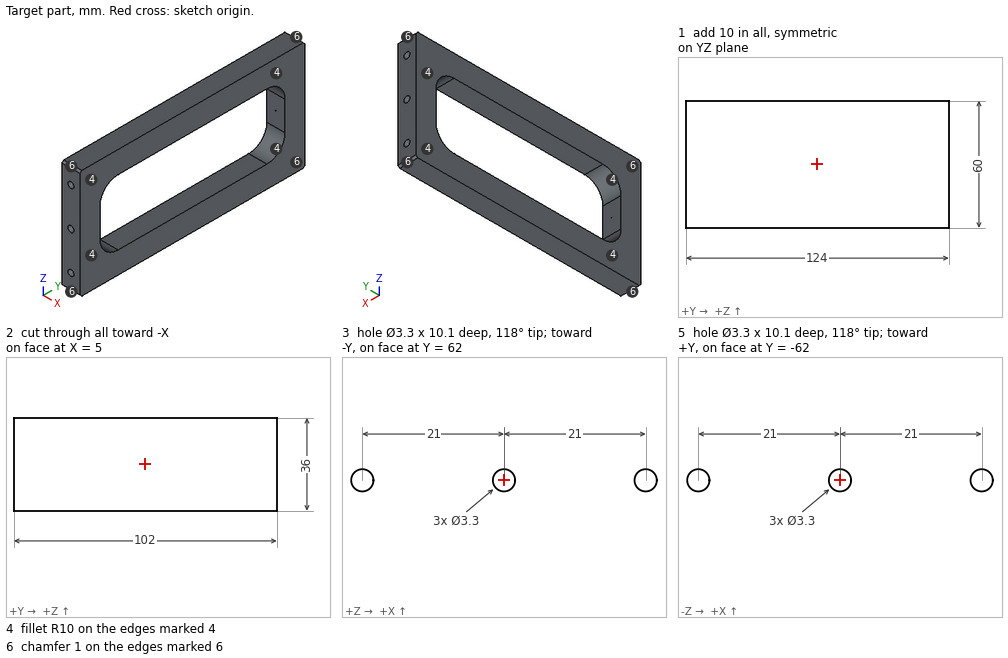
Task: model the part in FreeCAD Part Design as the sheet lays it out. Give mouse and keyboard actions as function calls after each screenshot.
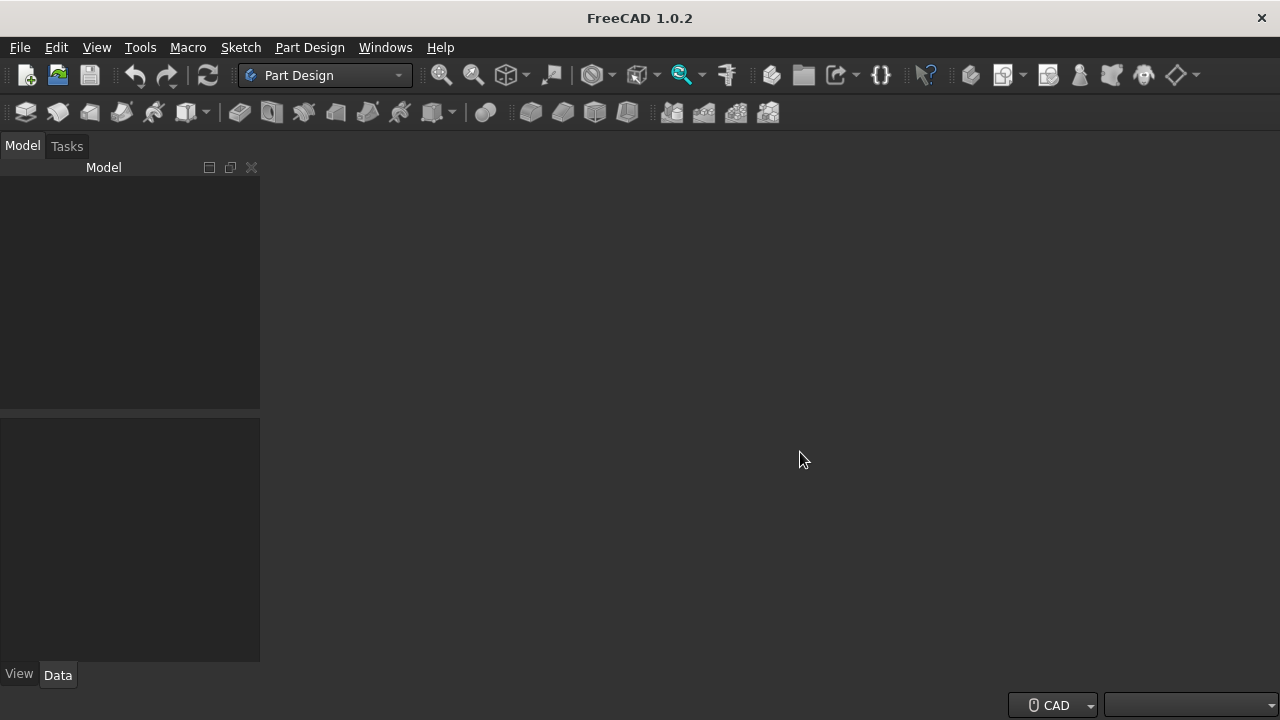
key(ctrl+n)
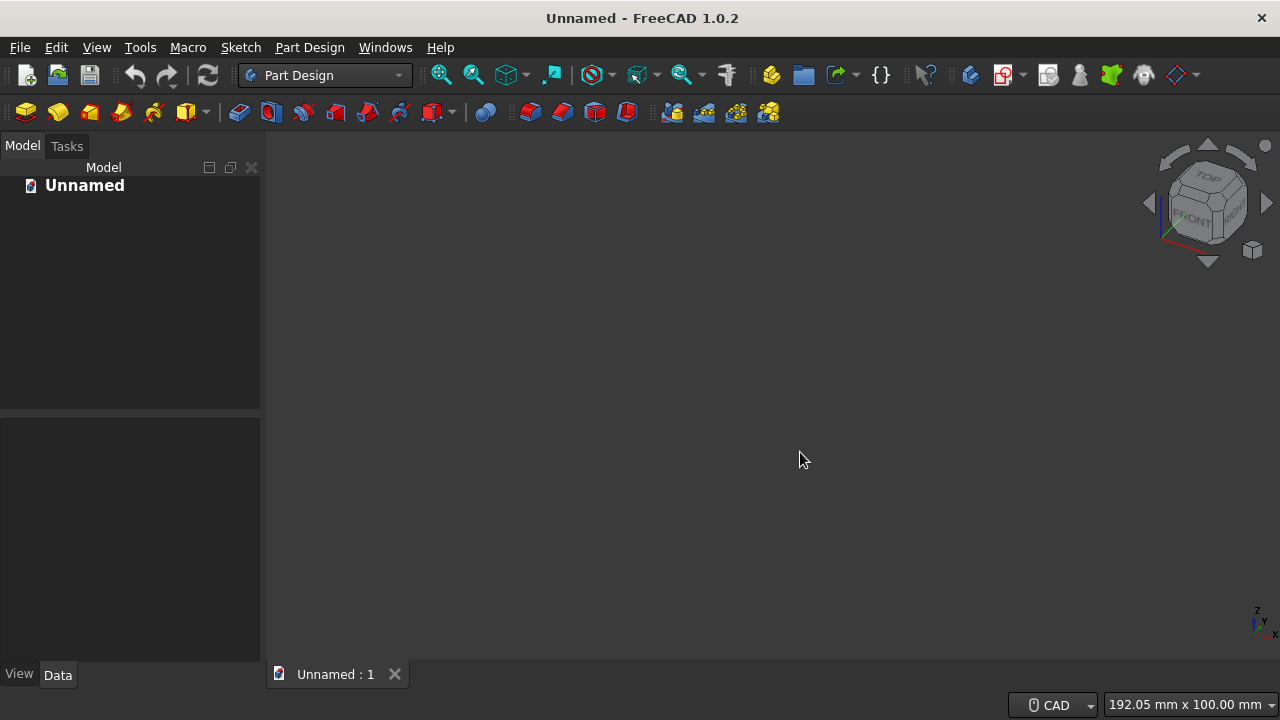
click(1004, 76)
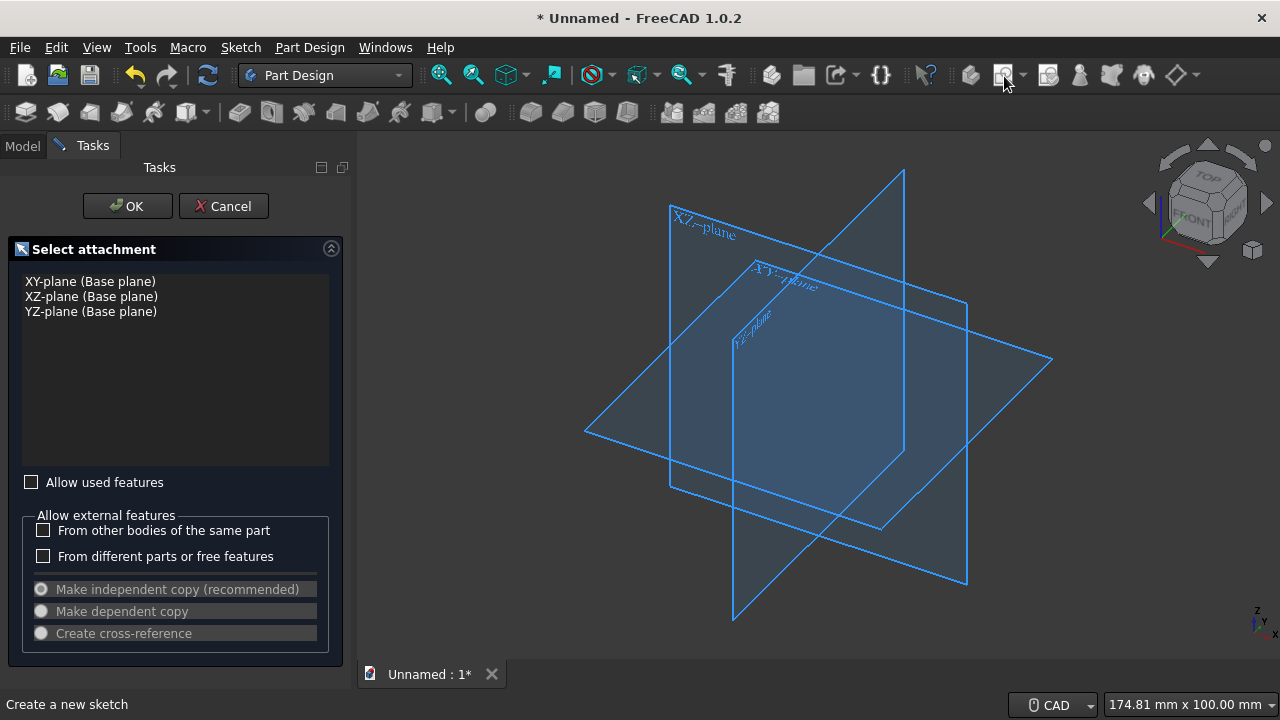
click(82, 312)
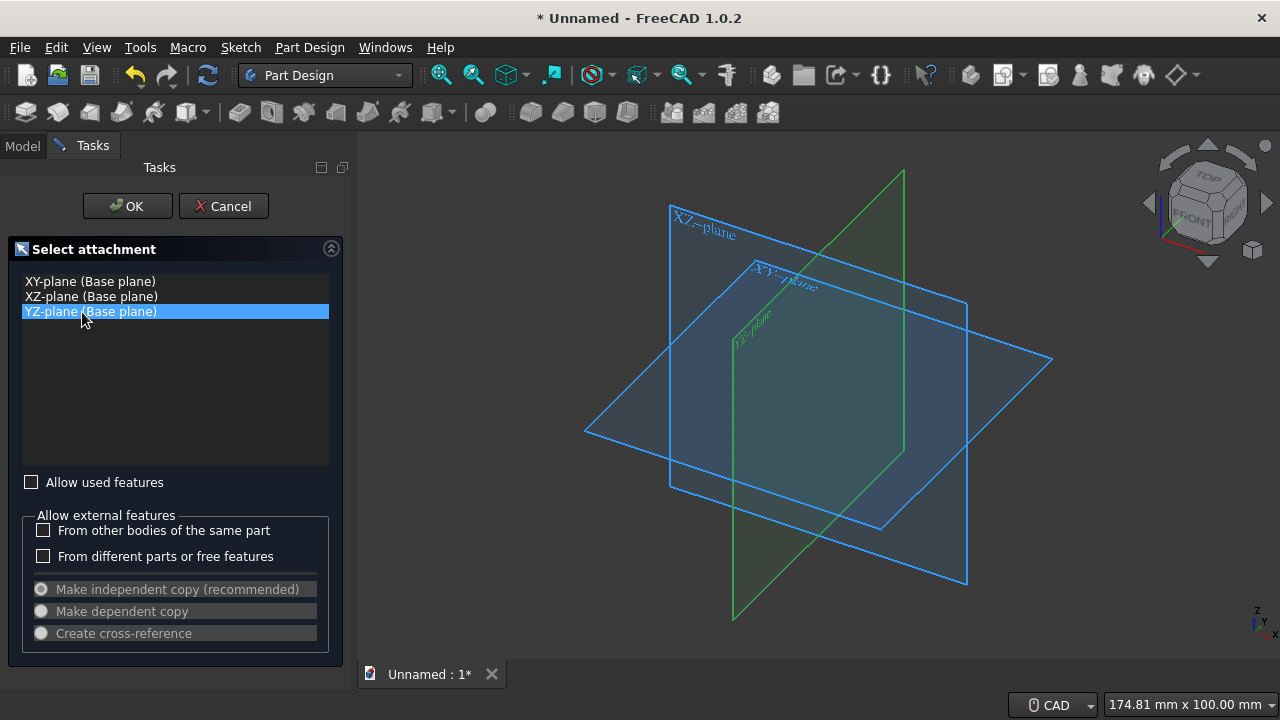
click(128, 206)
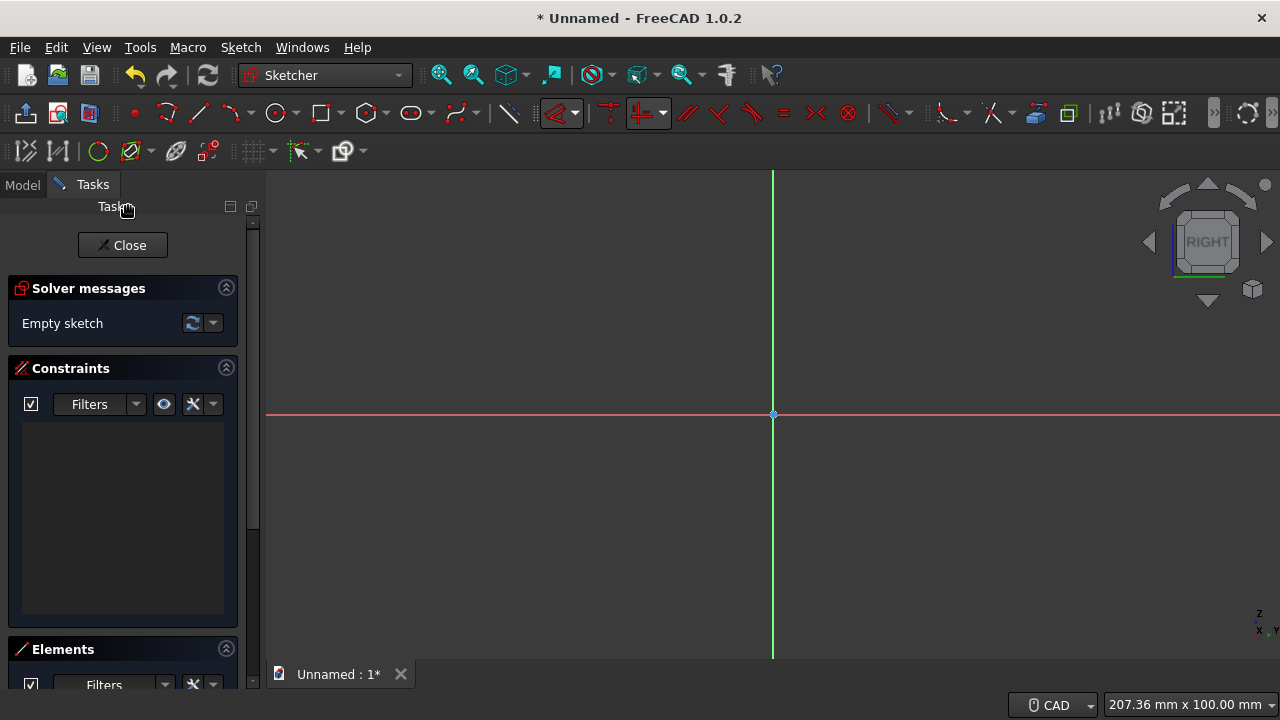
key(g)
key(v)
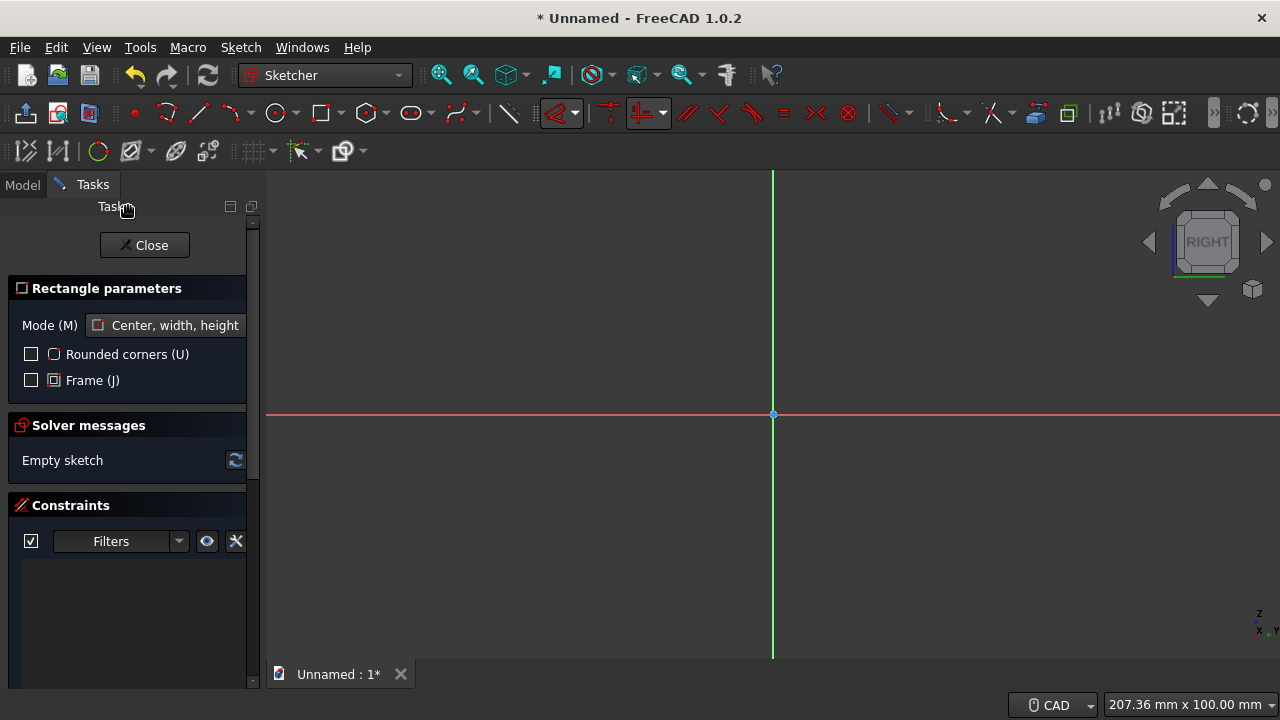
click(773, 414)
move(1076, 268)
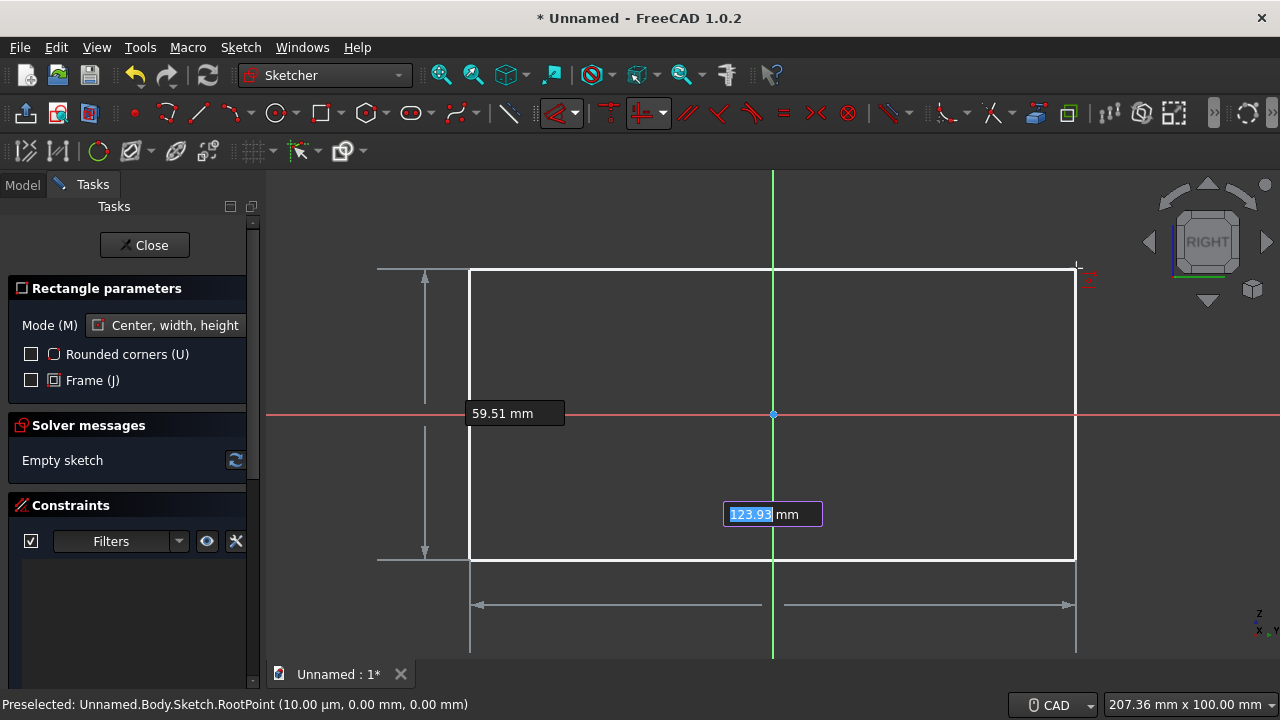
text(124)
key(Tab)
text(60)
key(Return)
key(Escape)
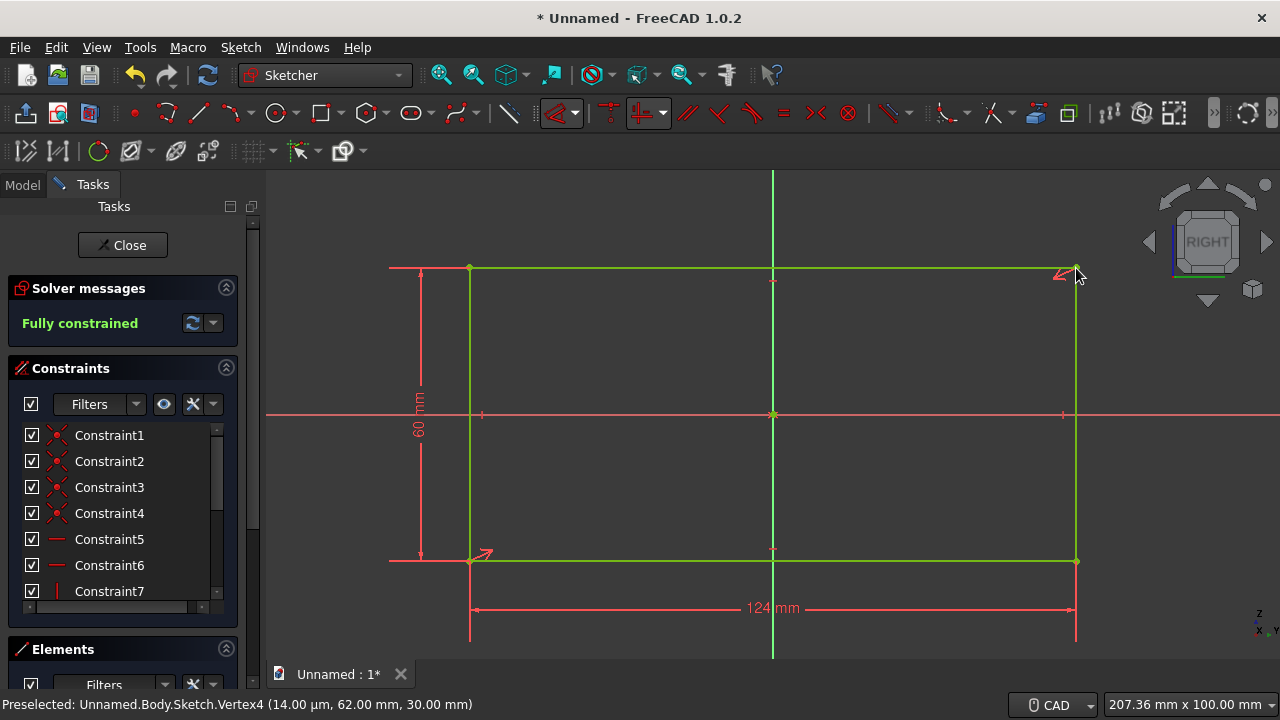
click(123, 245)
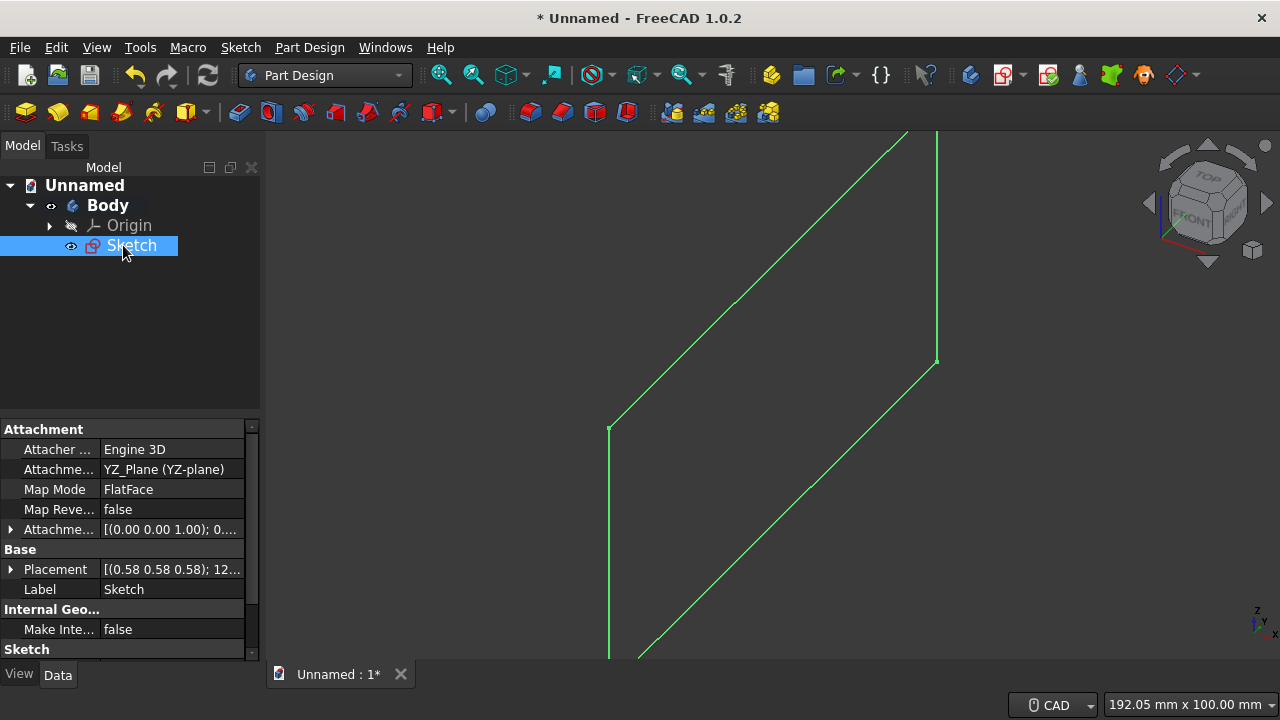
click(26, 112)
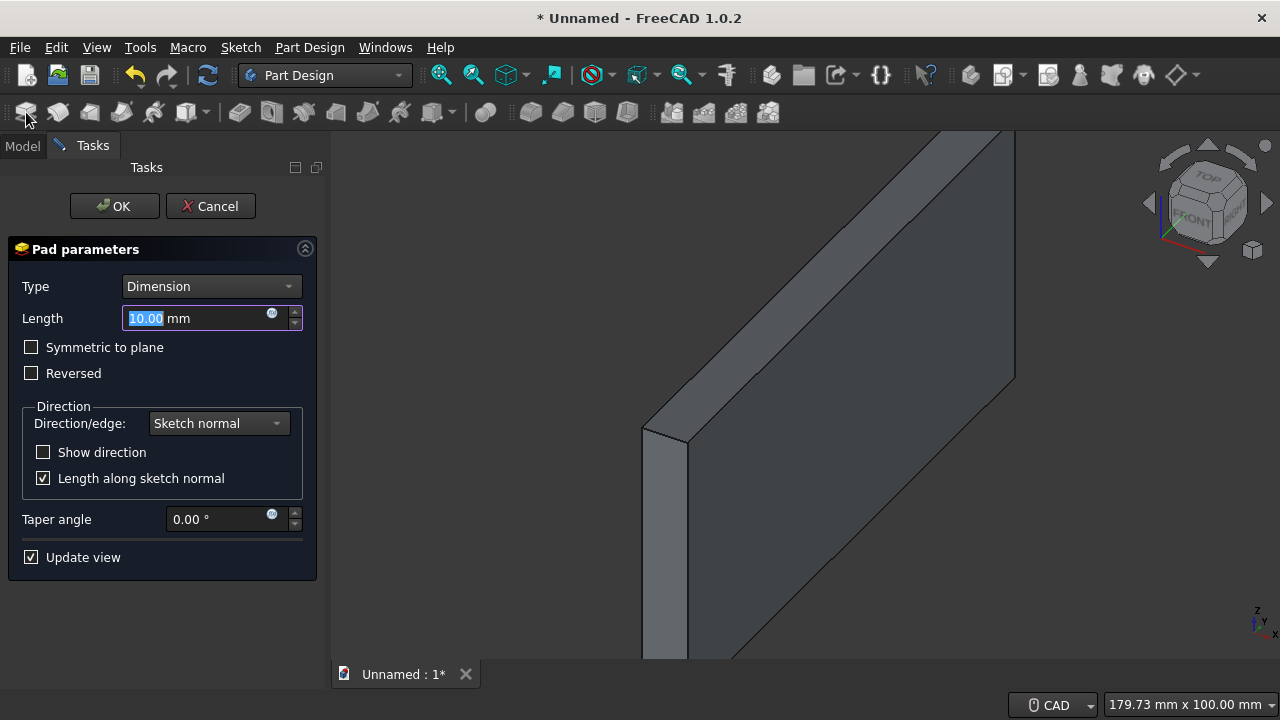
text(10)
key(Tab)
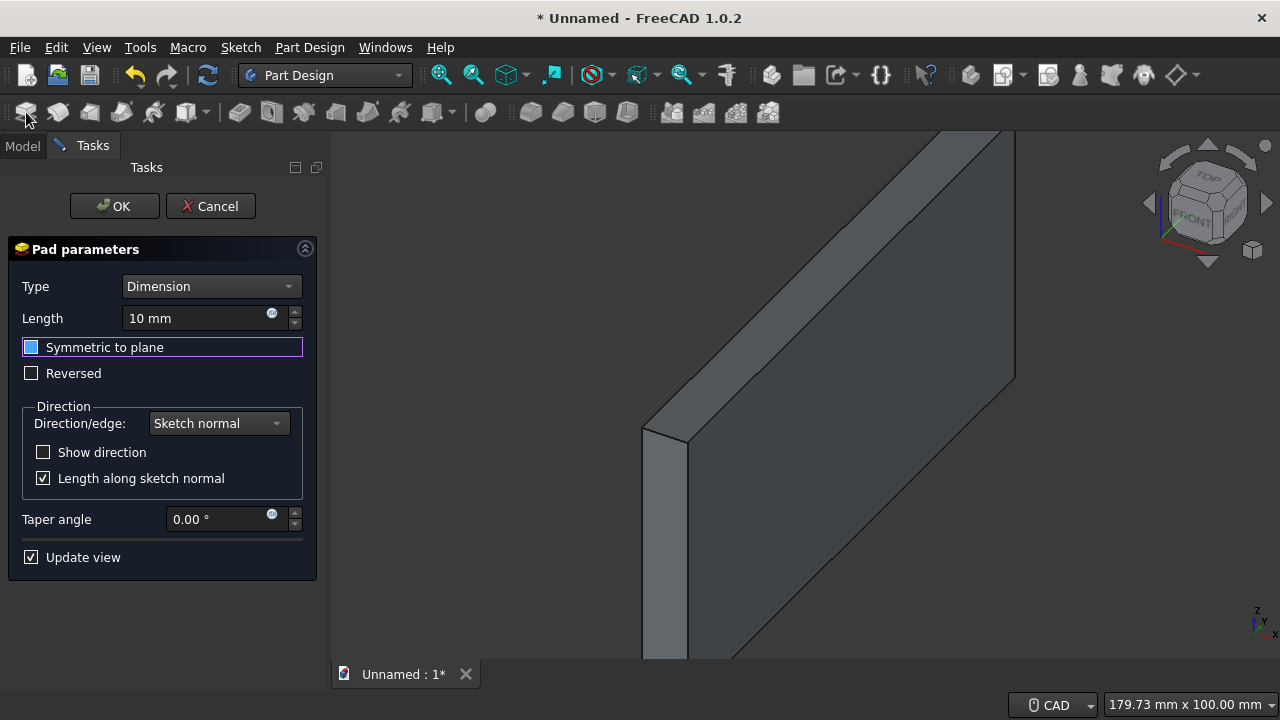
click(30, 347)